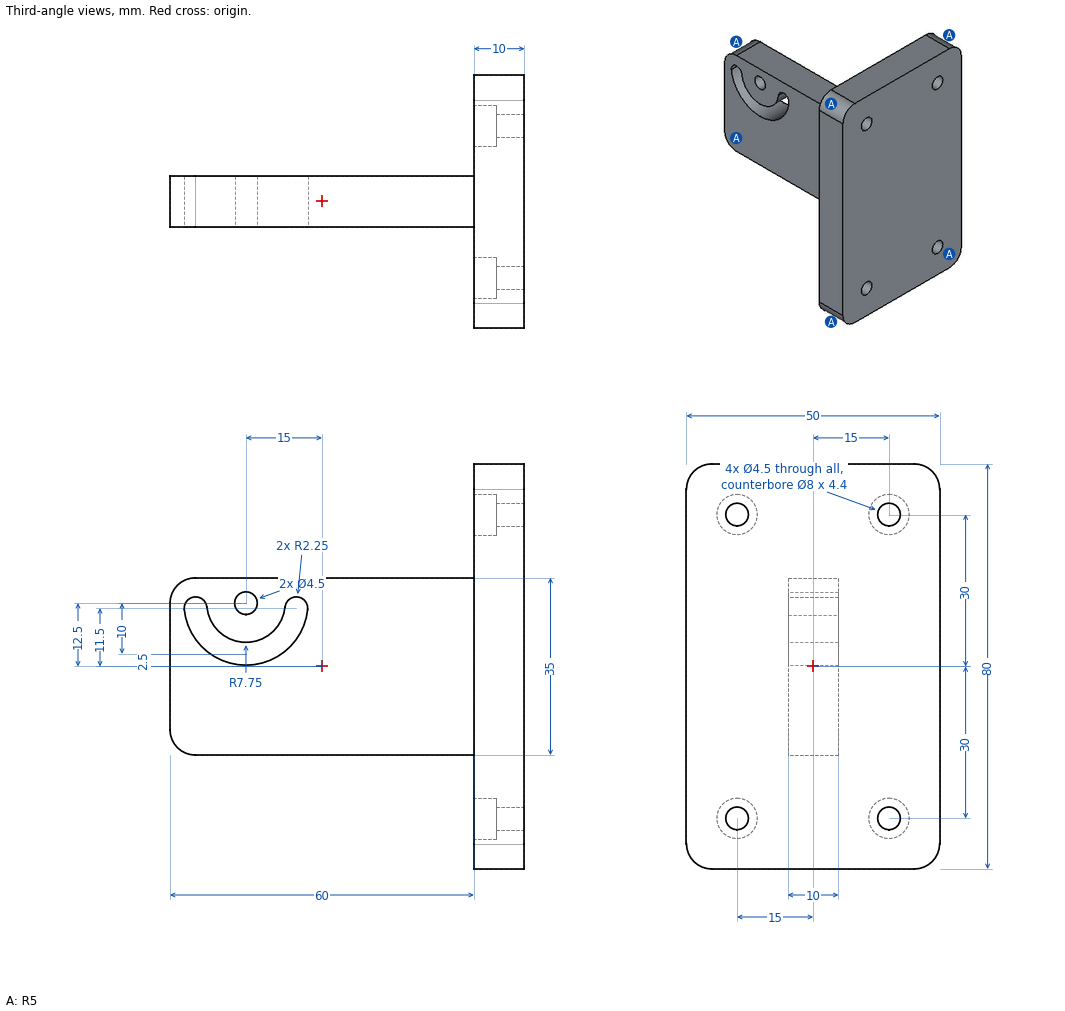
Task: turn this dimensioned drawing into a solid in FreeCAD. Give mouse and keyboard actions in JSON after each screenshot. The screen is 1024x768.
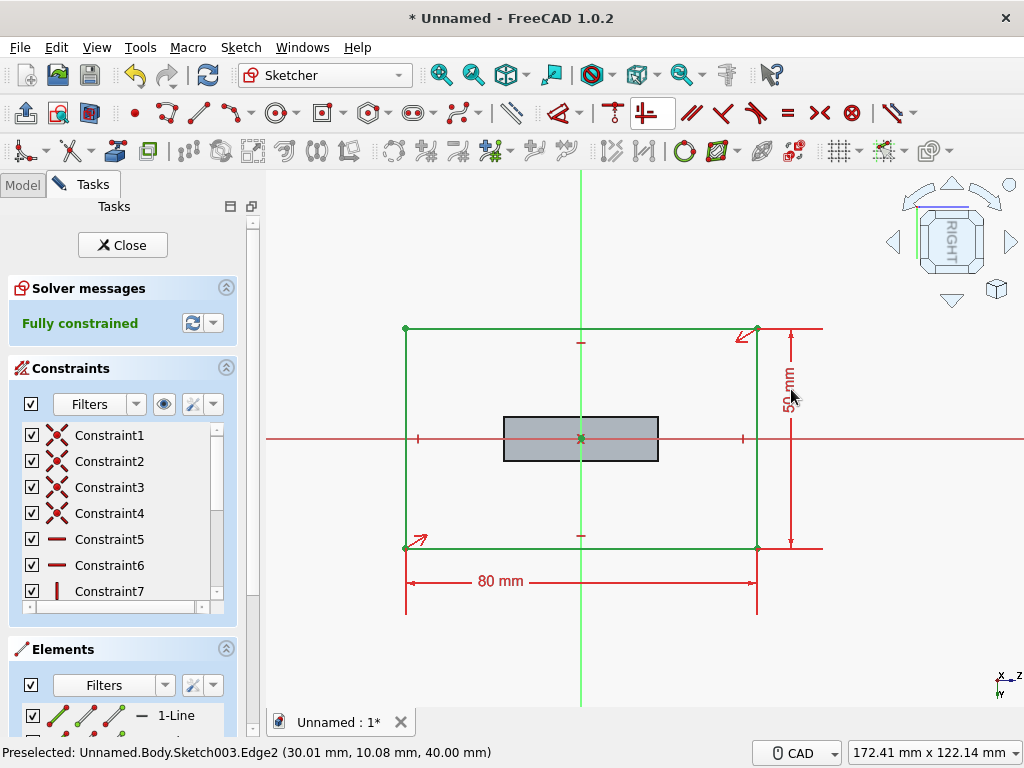
{"action": "left_click", "coordinate": [123, 245]}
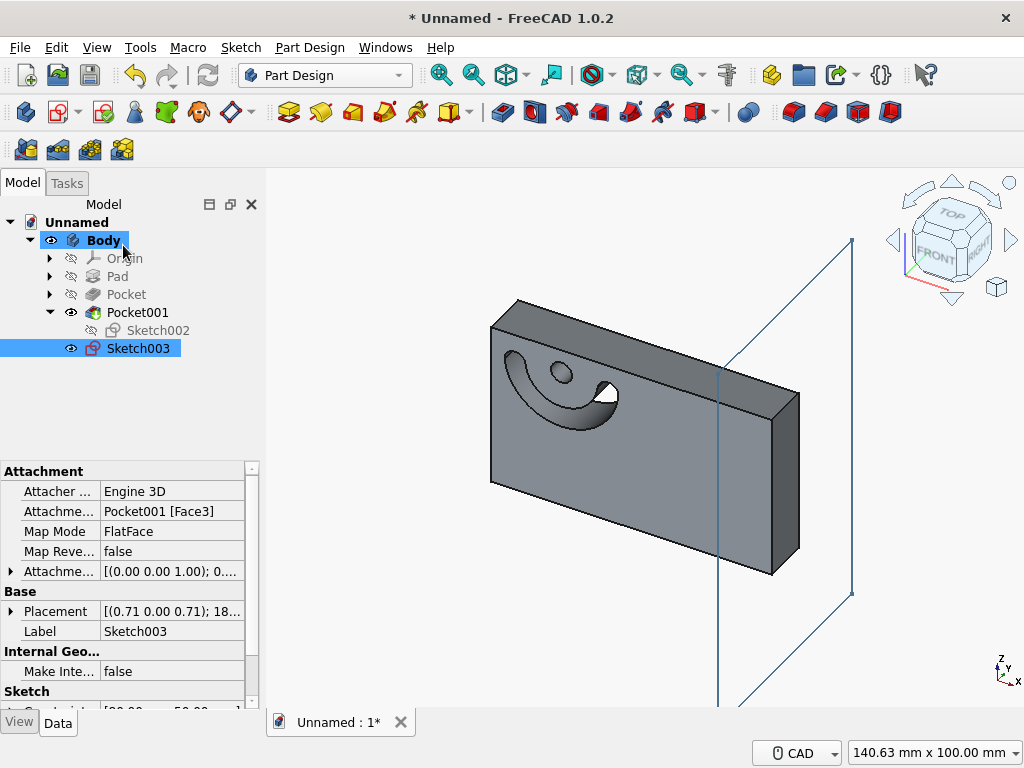
{"action": "left_click", "coordinate": [290, 112]}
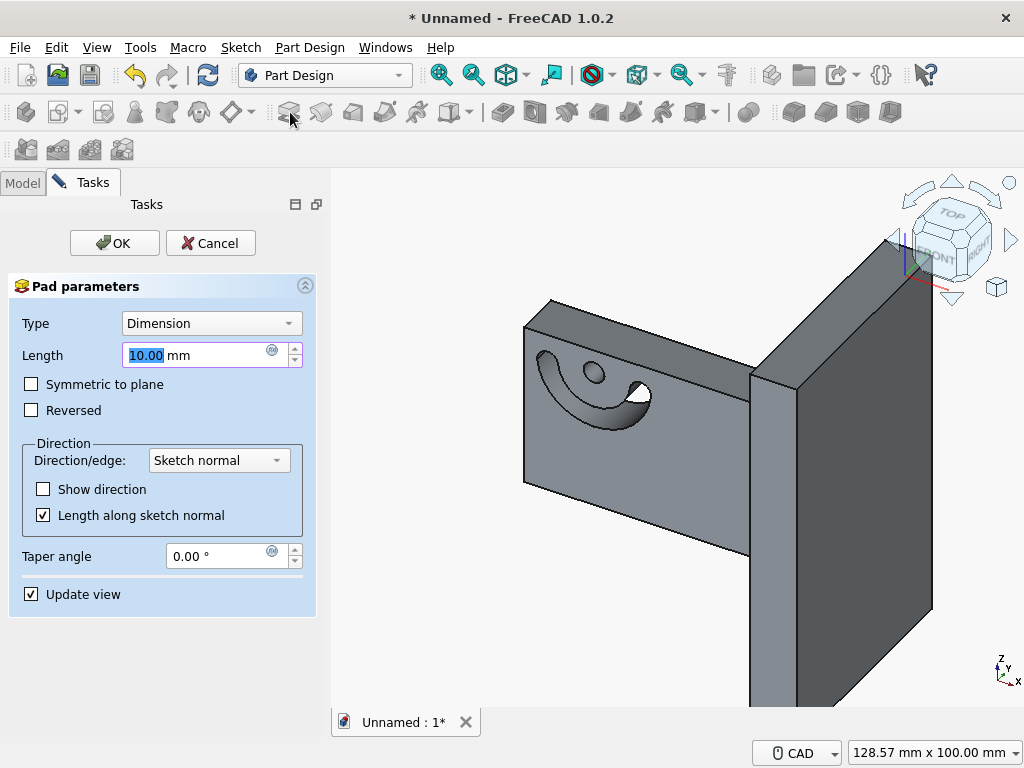
{"action": "type", "text": "10"}
{"action": "key", "text": "Tab"}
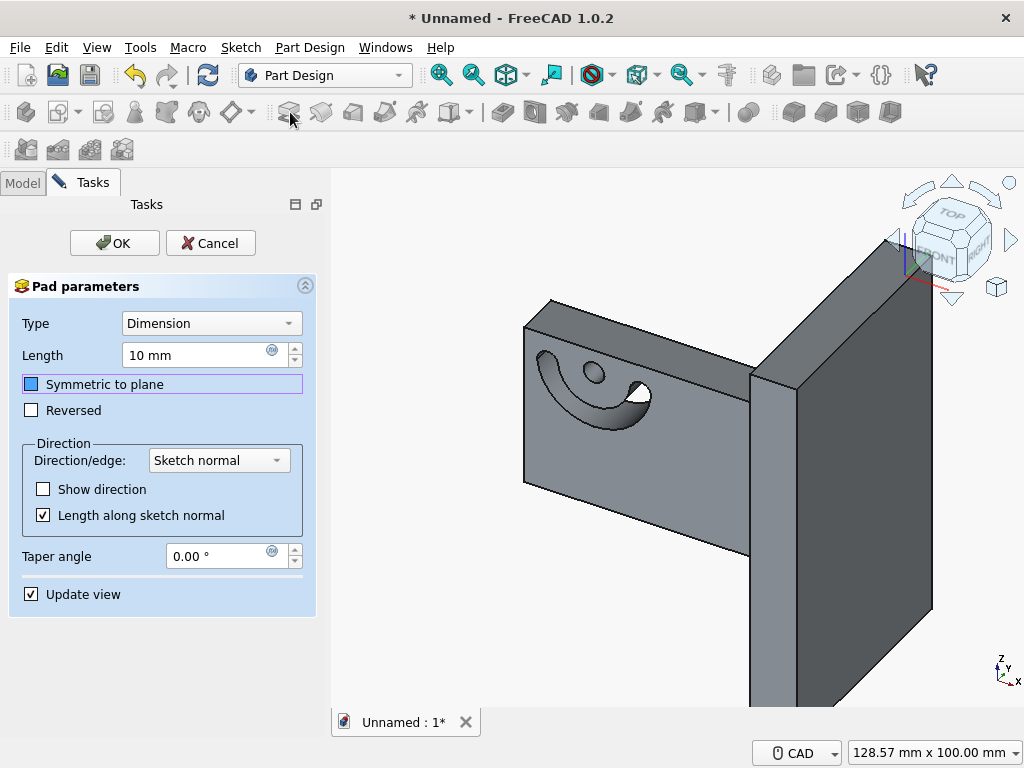
{"action": "left_click", "coordinate": [115, 243]}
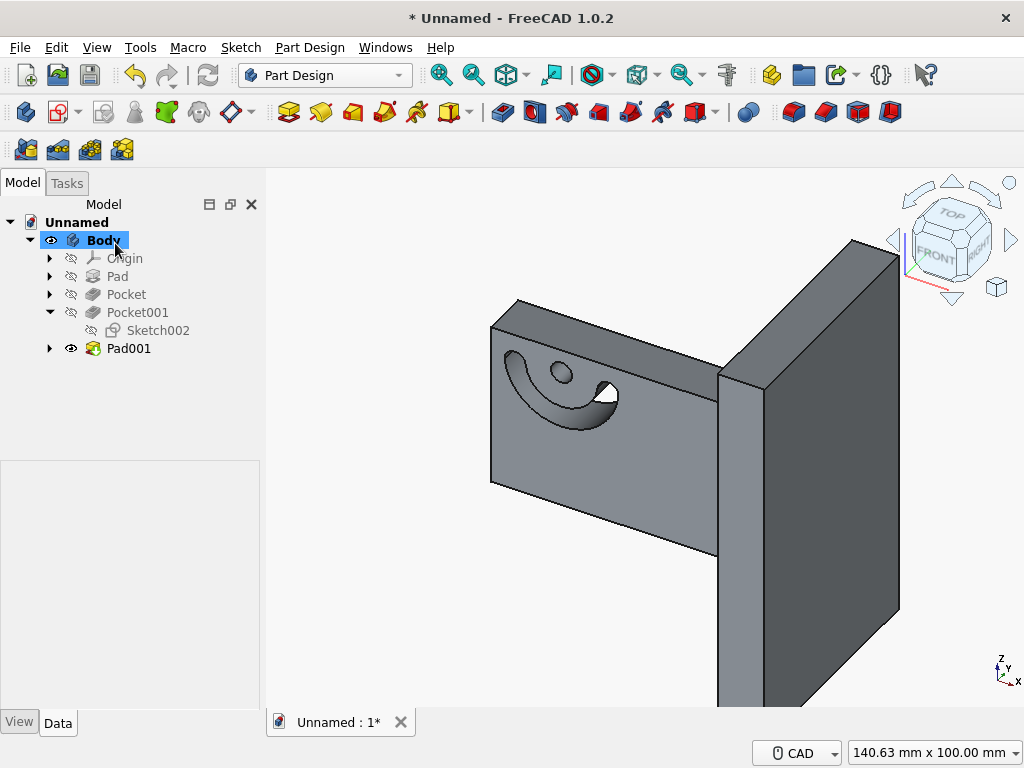
{"action": "left_click", "coordinate": [442, 76]}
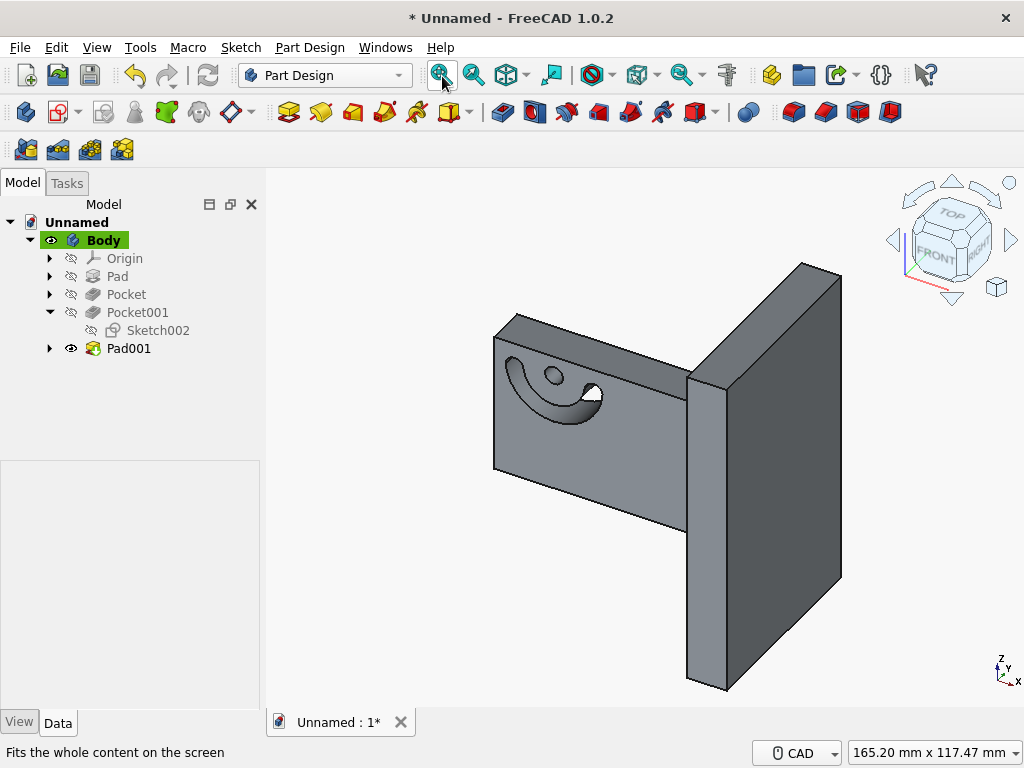
{"action": "key", "text": "6"}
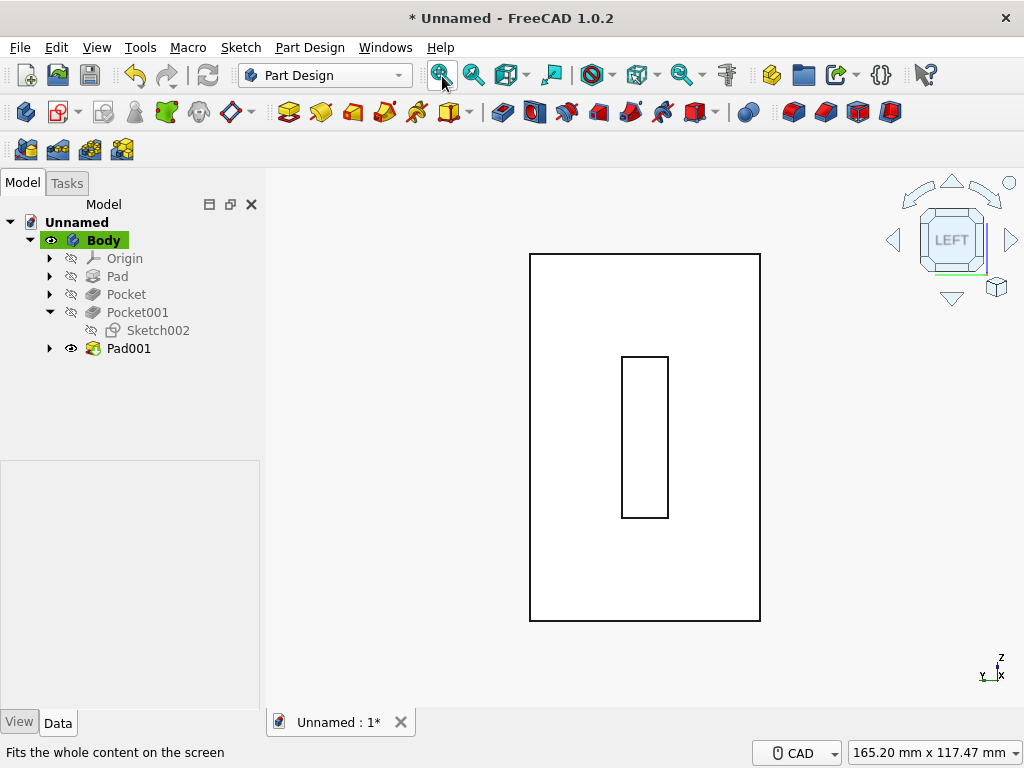
{"action": "left_click", "coordinate": [711, 332]}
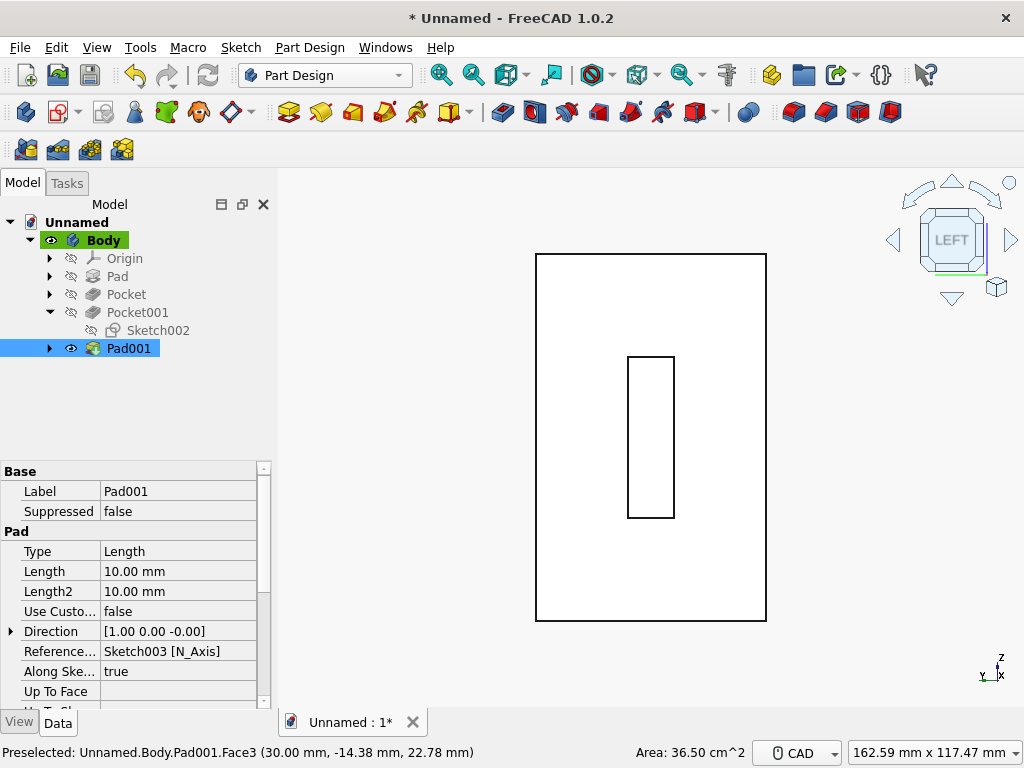
{"action": "left_click", "coordinate": [58, 112]}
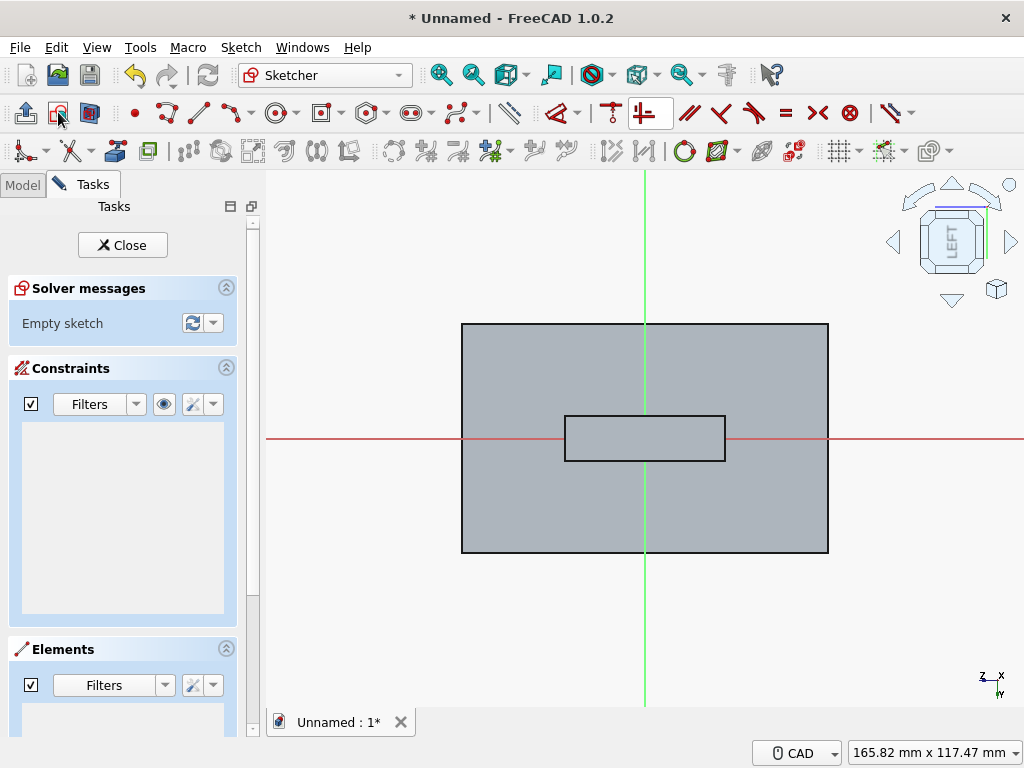
{"action": "scroll", "coordinate": [784, 439], "scroll_direction": "up", "scroll_amount": 2}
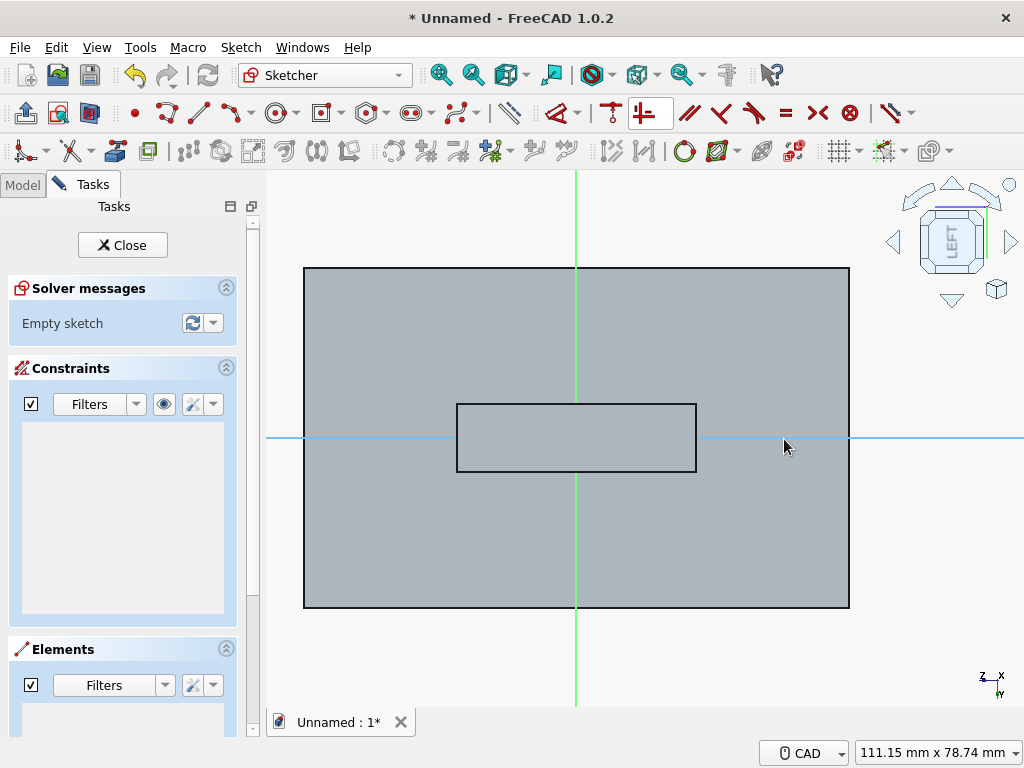
{"action": "left_click", "coordinate": [276, 114]}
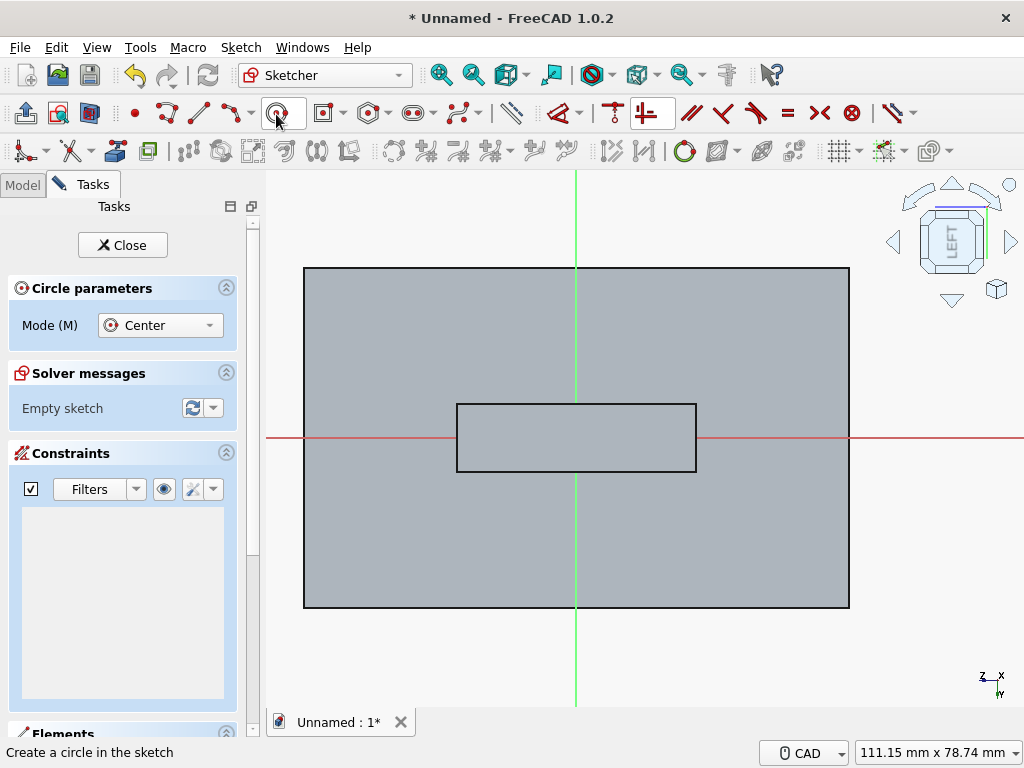
{"action": "scroll", "coordinate": [372, 540], "scroll_direction": "up", "scroll_amount": 2}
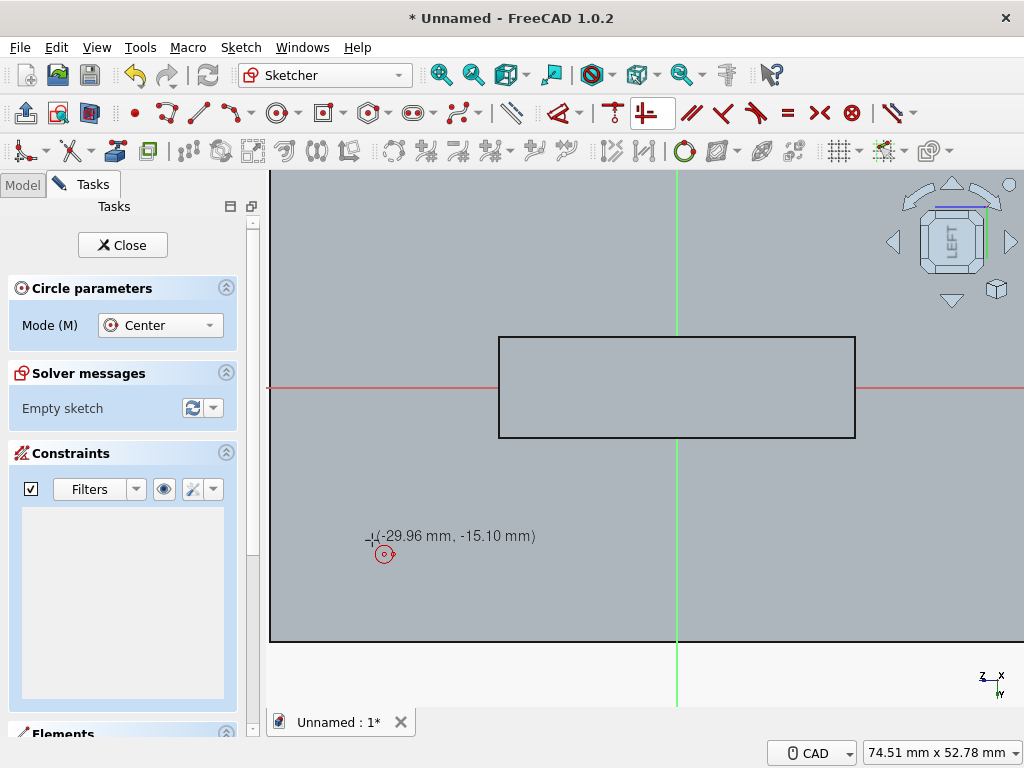
{"action": "left_click", "coordinate": [372, 540]}
{"action": "left_click", "coordinate": [388, 524]}